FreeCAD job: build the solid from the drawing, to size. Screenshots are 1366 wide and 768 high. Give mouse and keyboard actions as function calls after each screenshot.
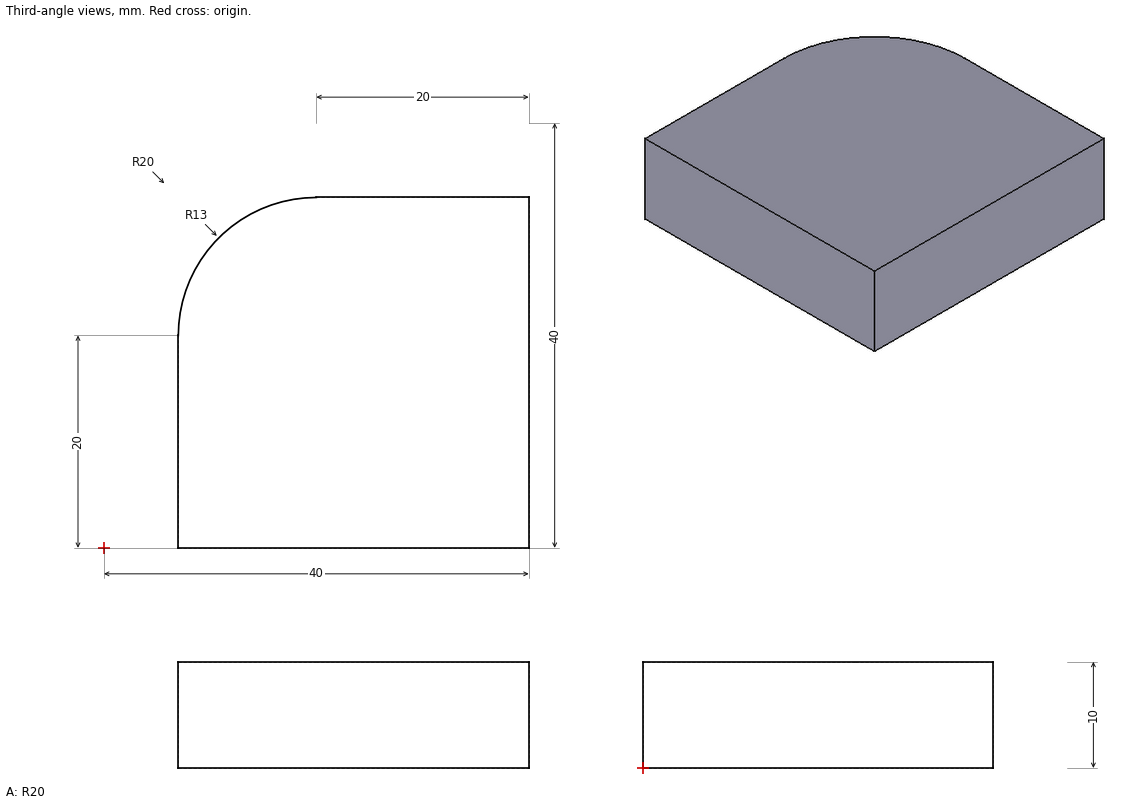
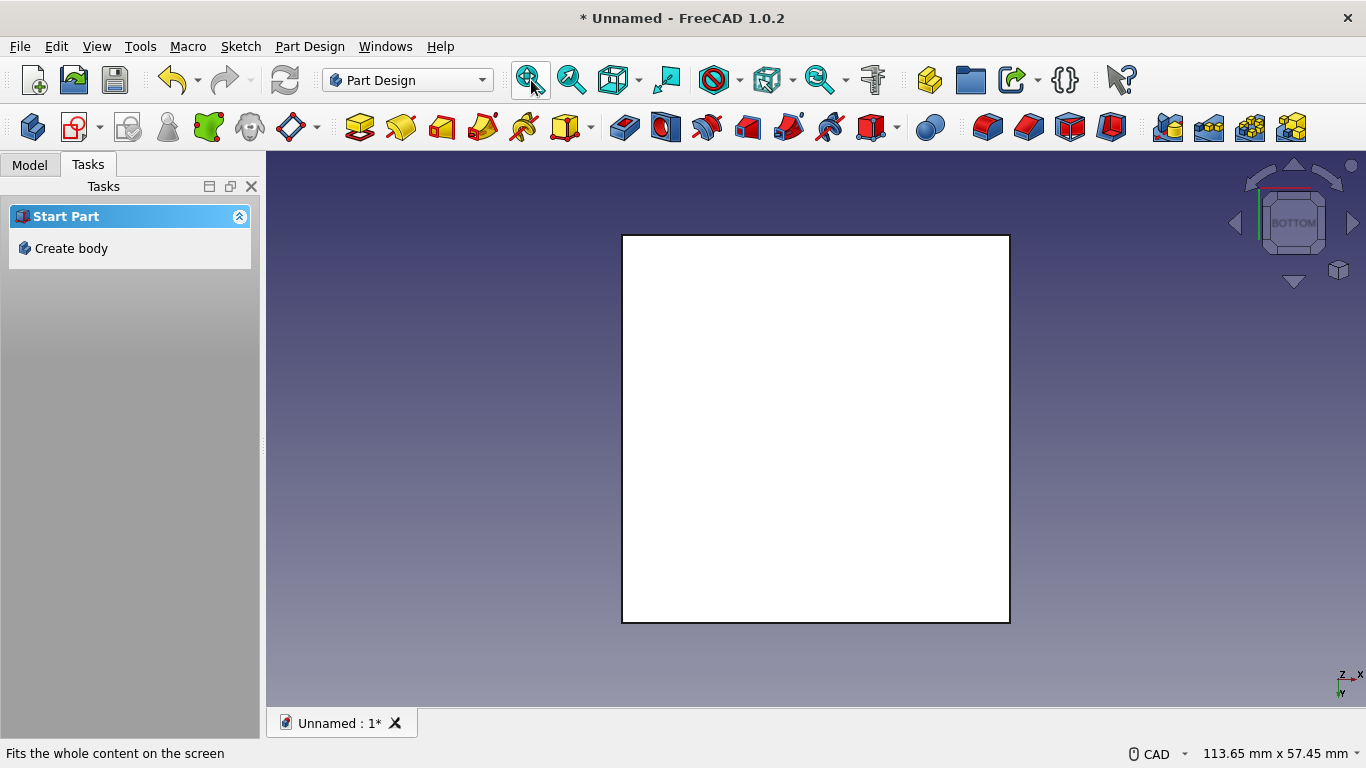
key(4)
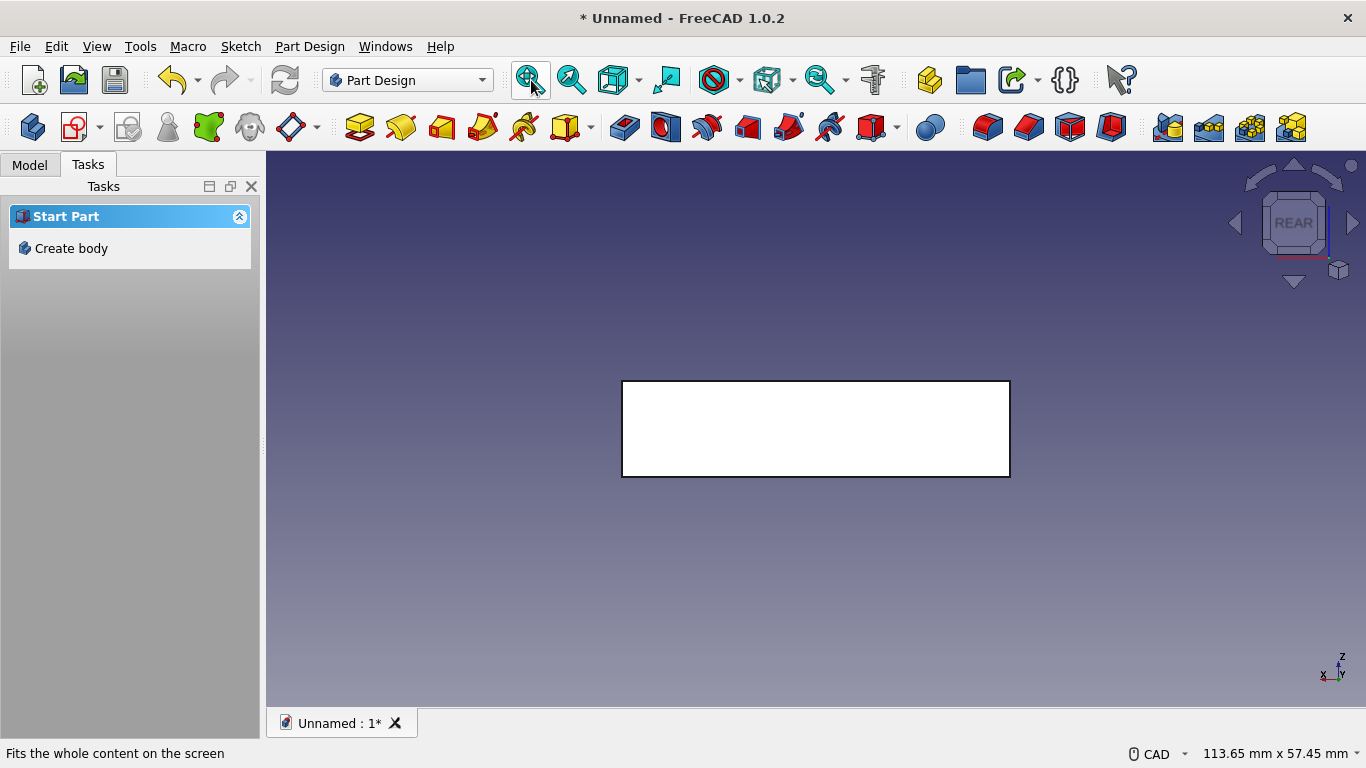
click(531, 80)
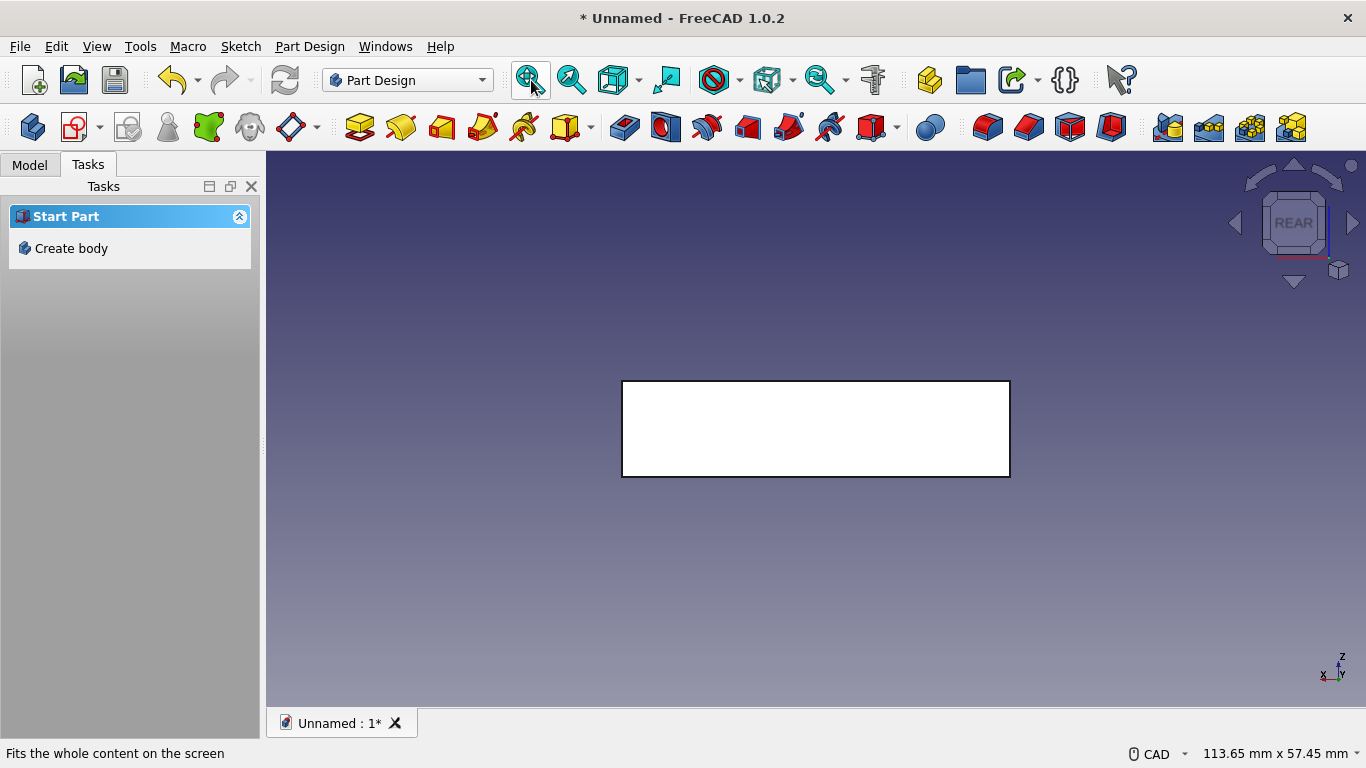
click(1010, 428)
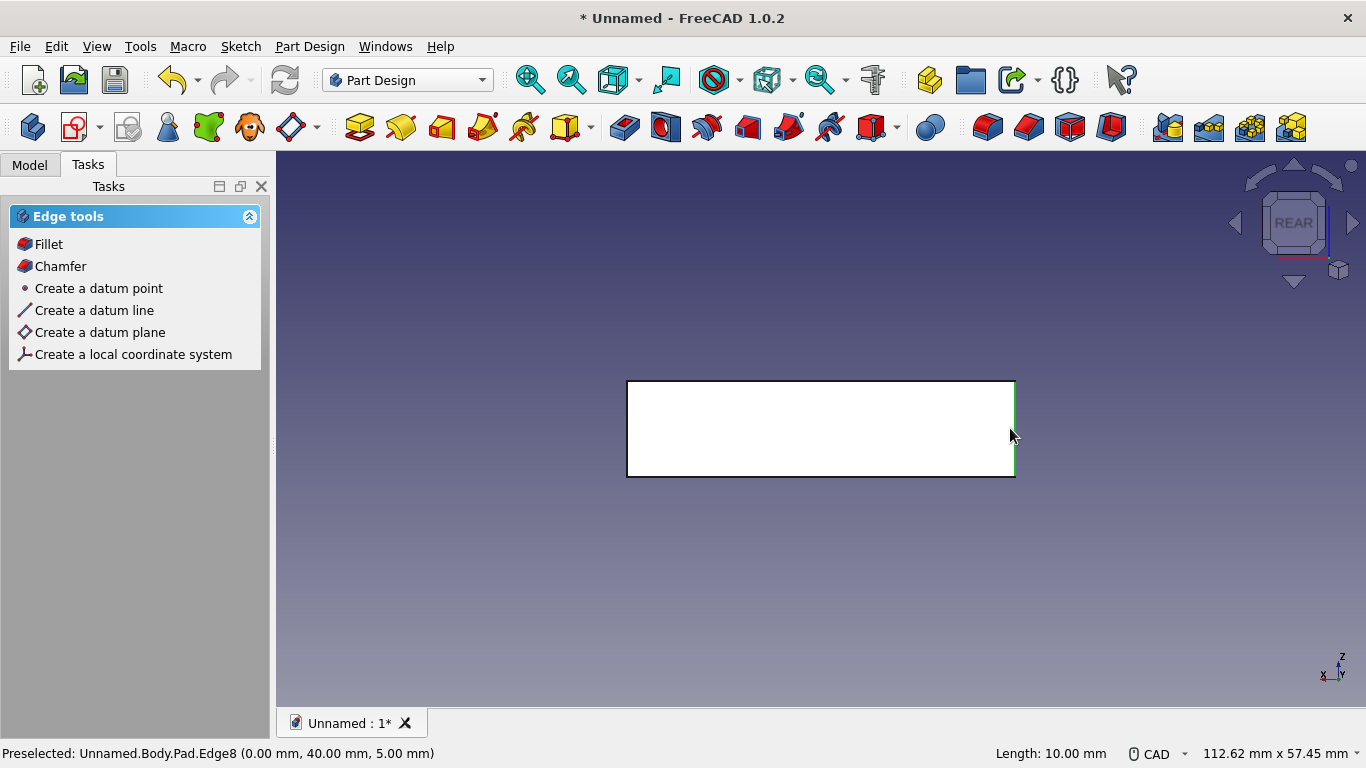
click(988, 128)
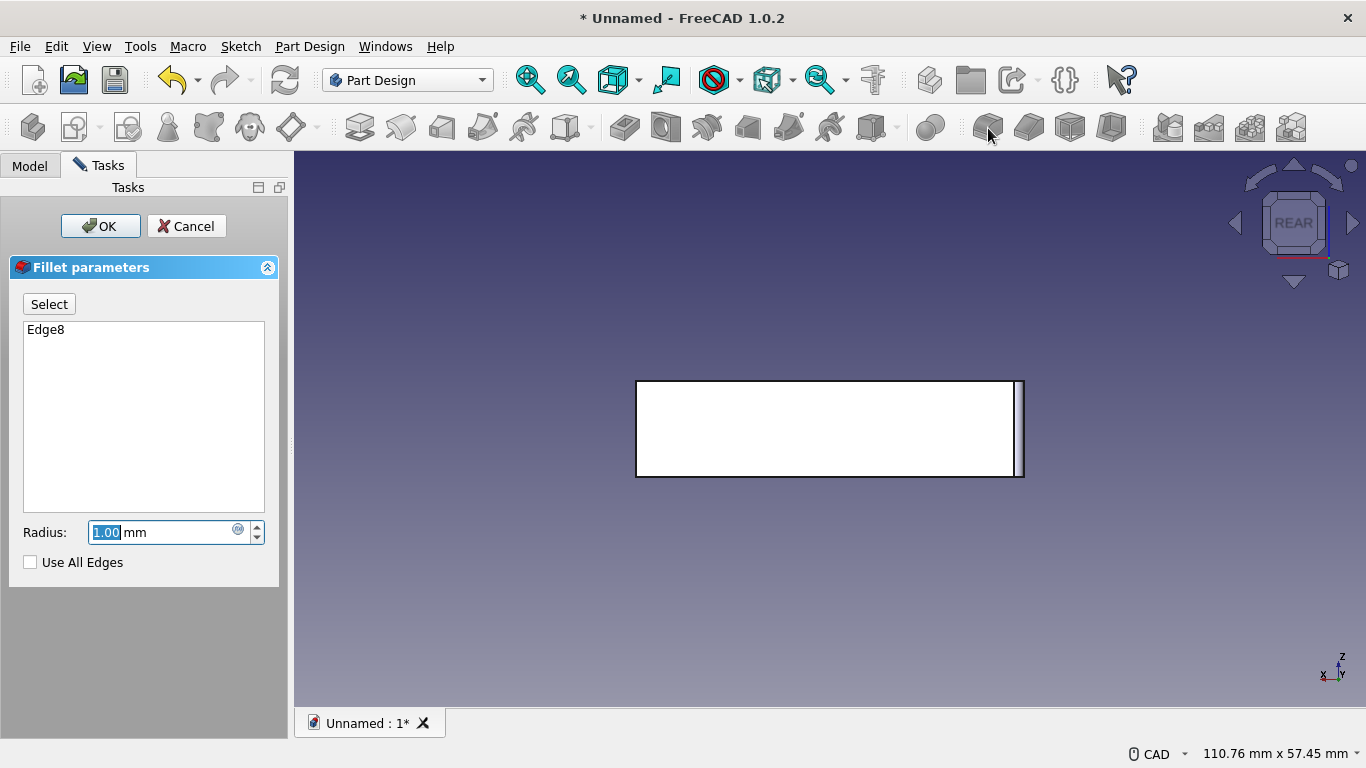
text(20)
key(Tab)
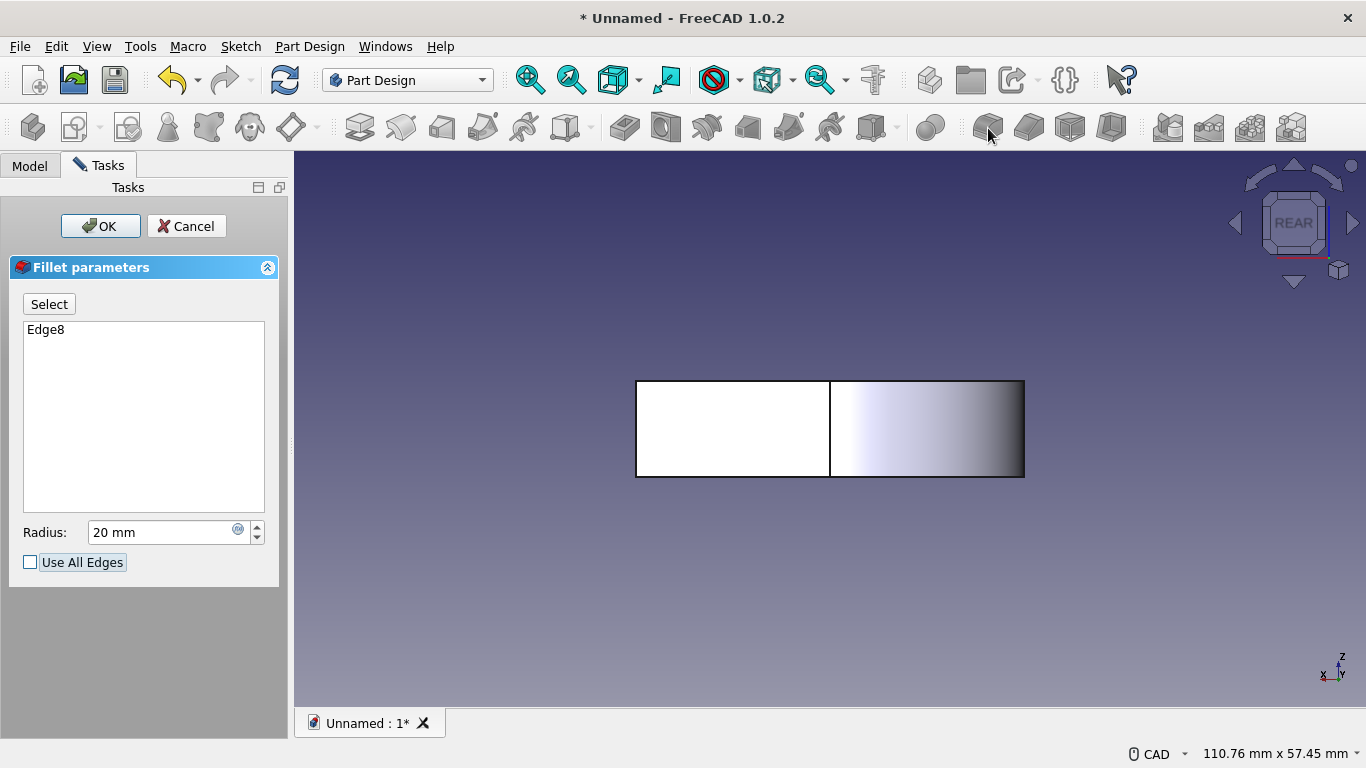
click(101, 226)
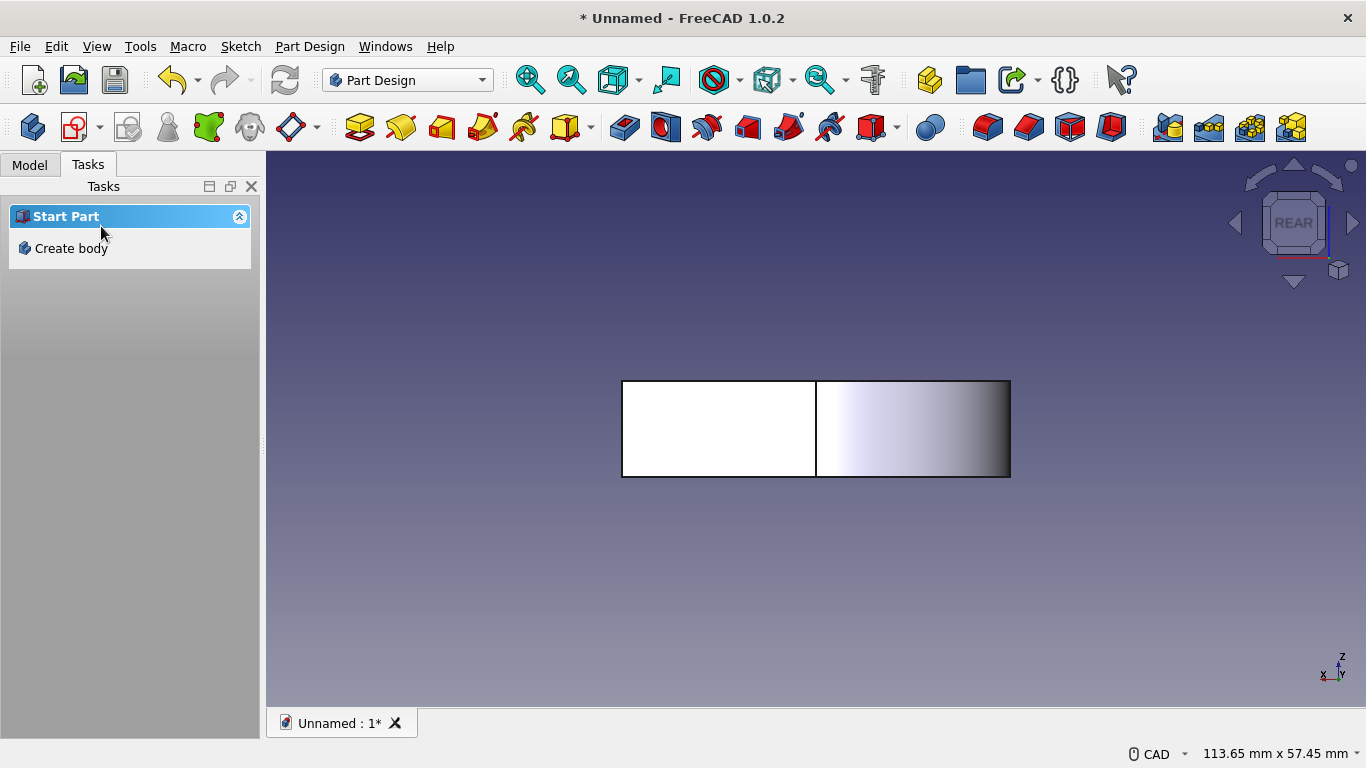
click(531, 80)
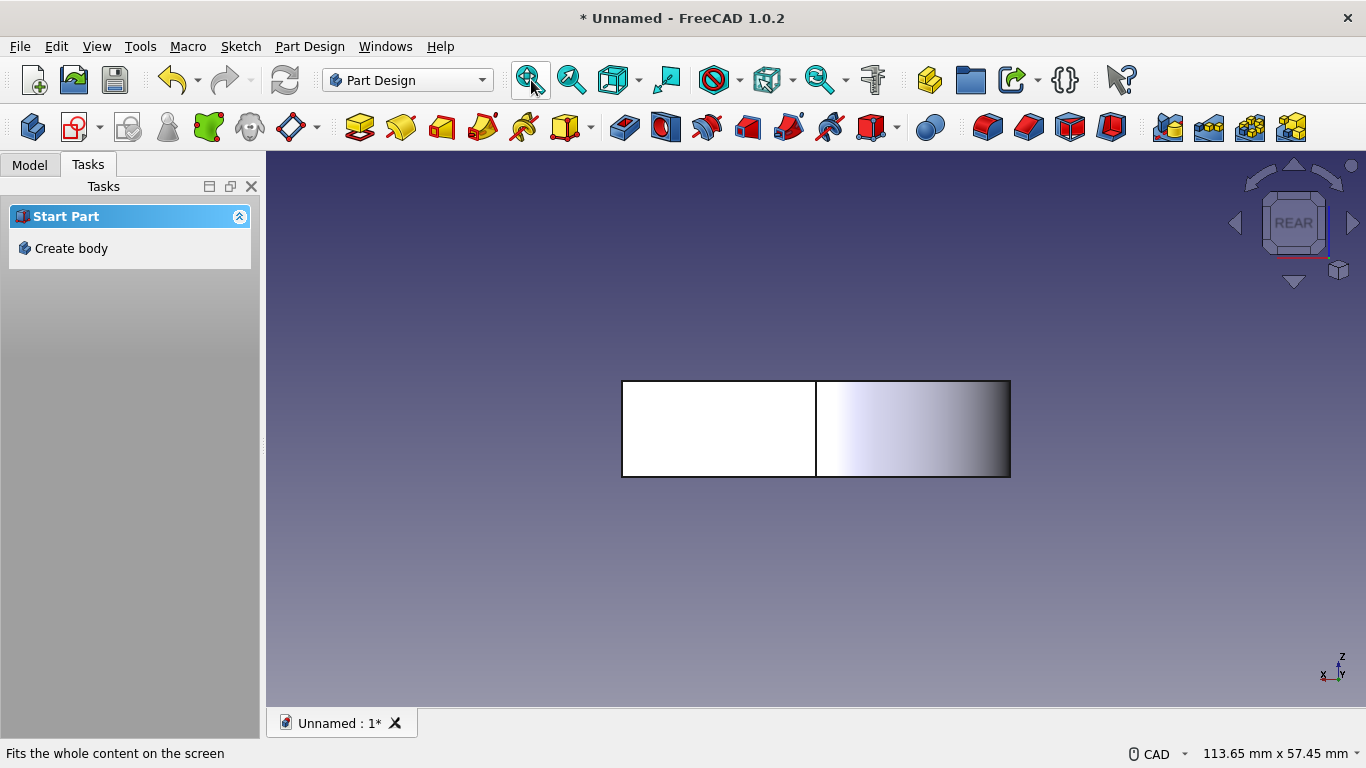
click(74, 128)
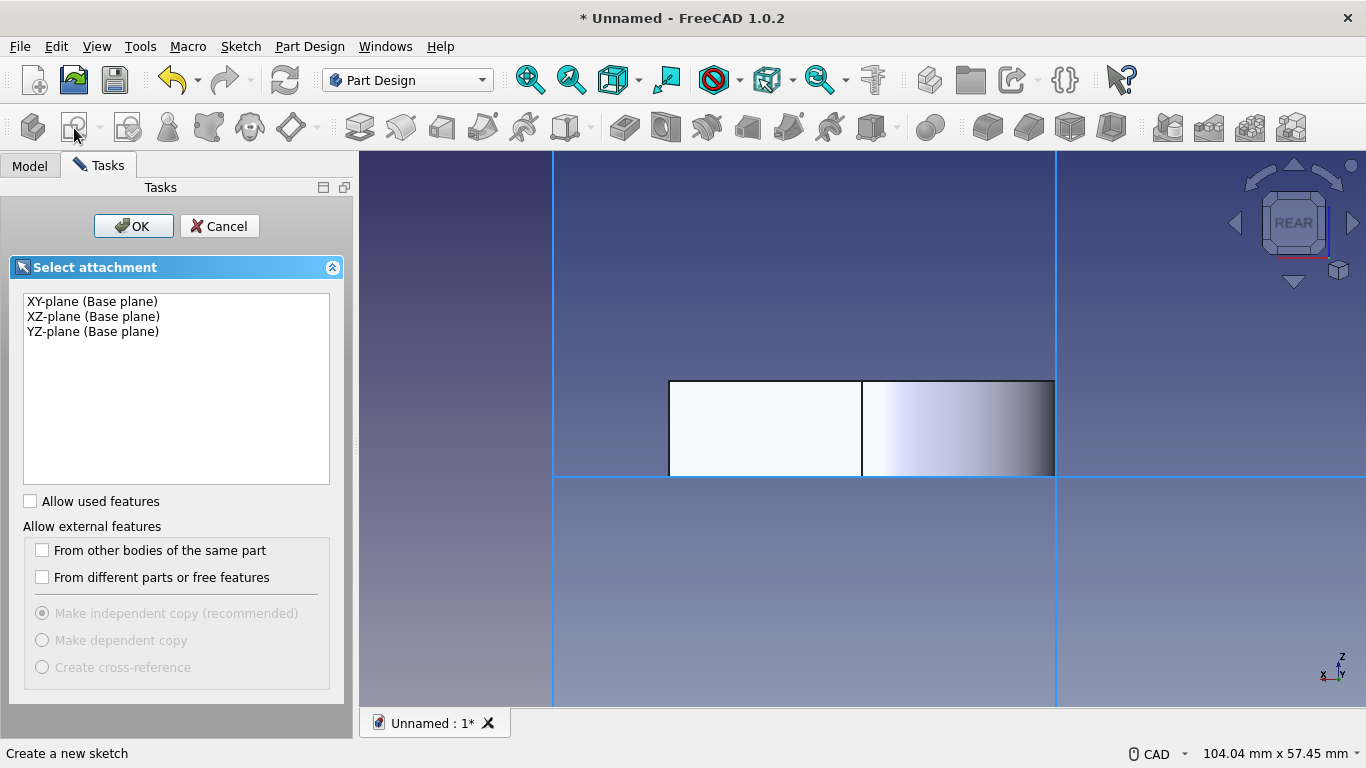
click(84, 302)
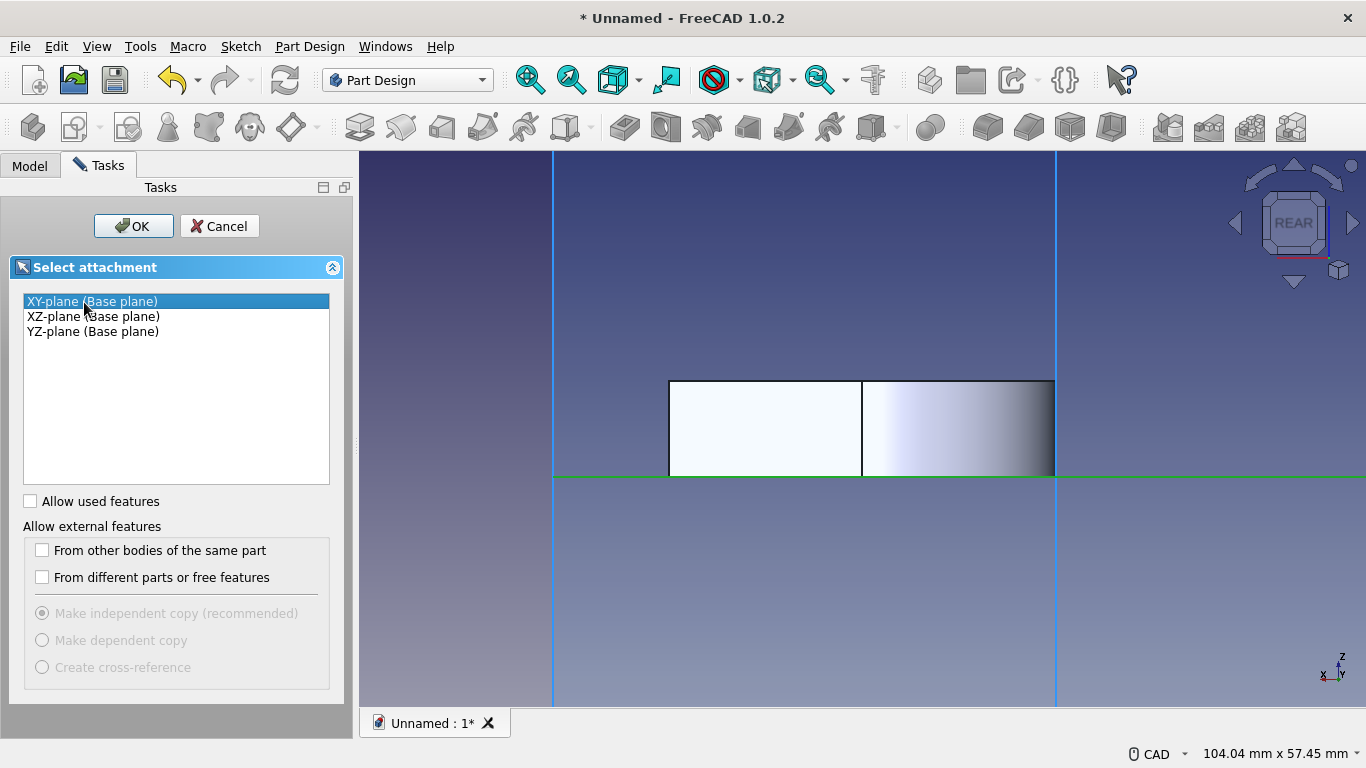
click(134, 226)